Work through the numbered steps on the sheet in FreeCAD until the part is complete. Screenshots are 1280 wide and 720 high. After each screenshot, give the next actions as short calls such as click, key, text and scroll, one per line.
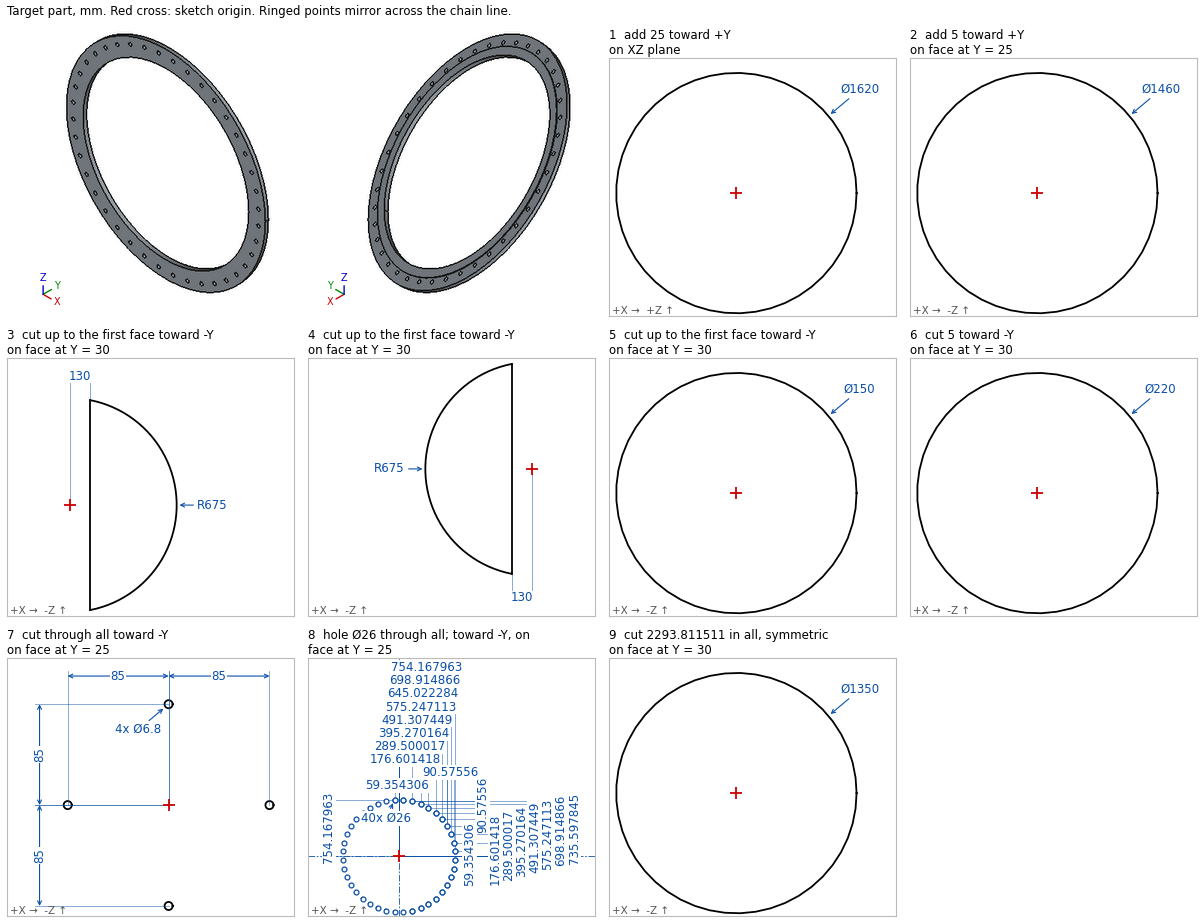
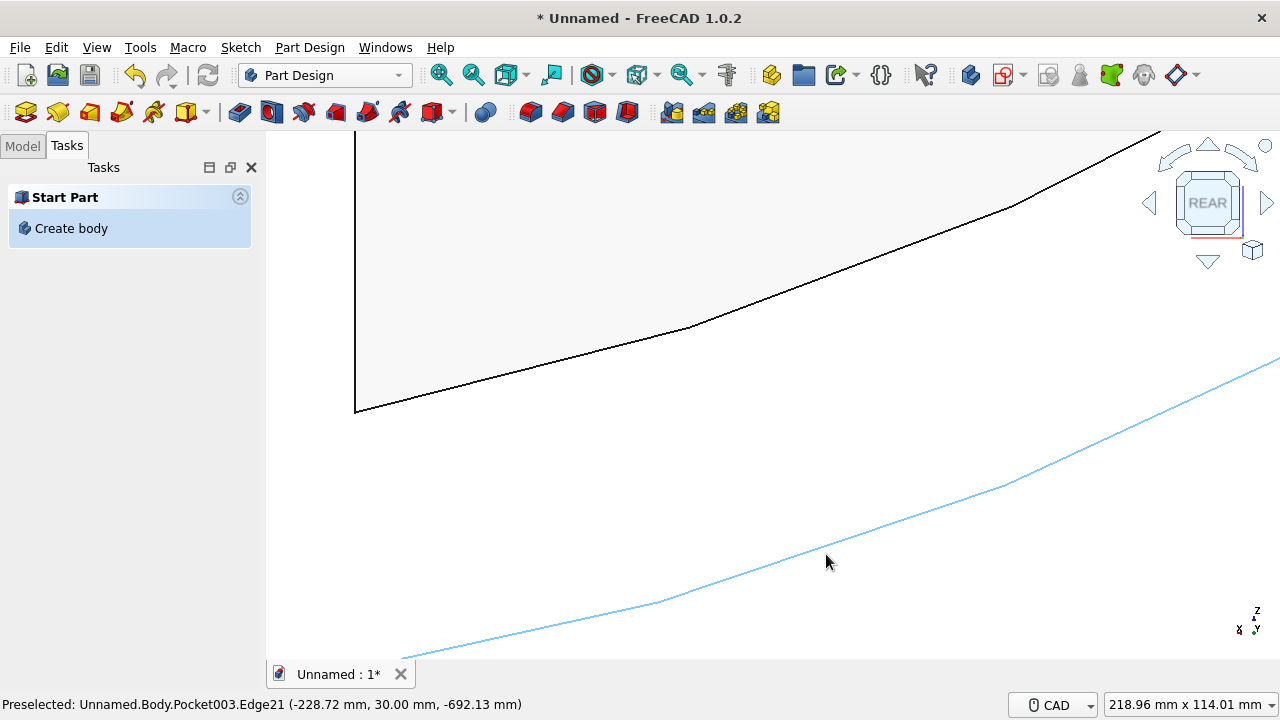
click(825, 559)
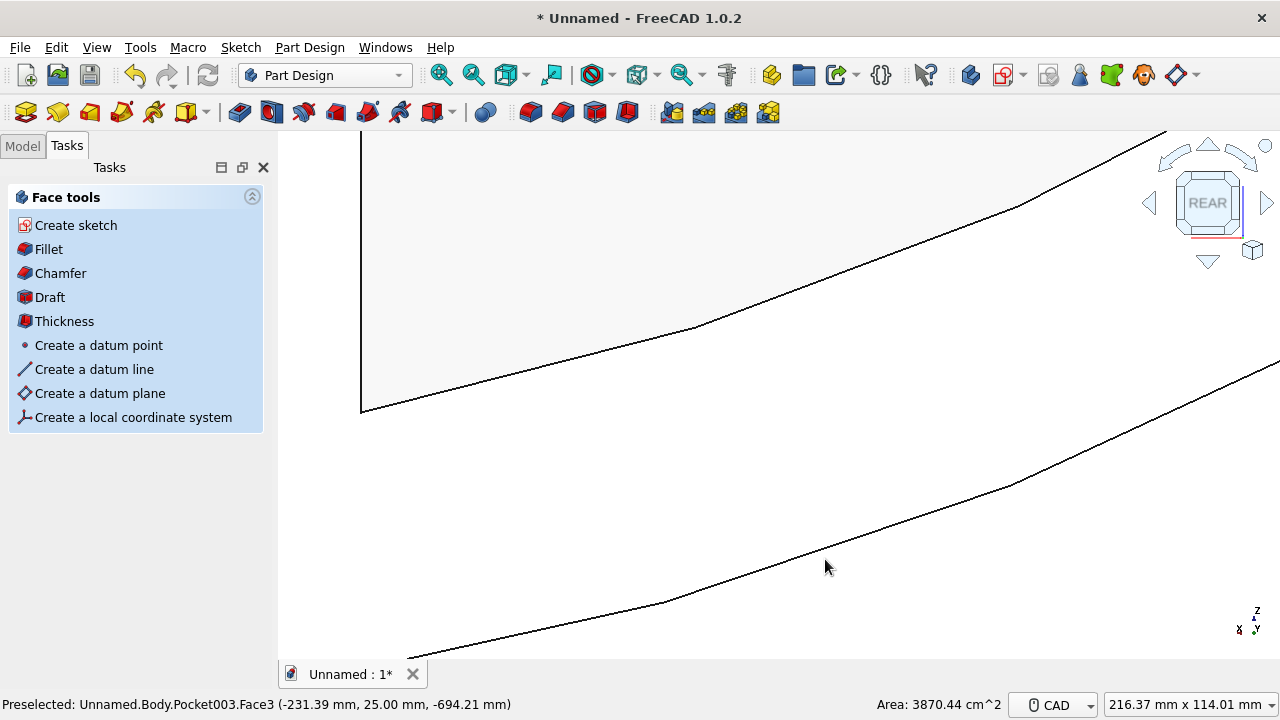
click(1004, 76)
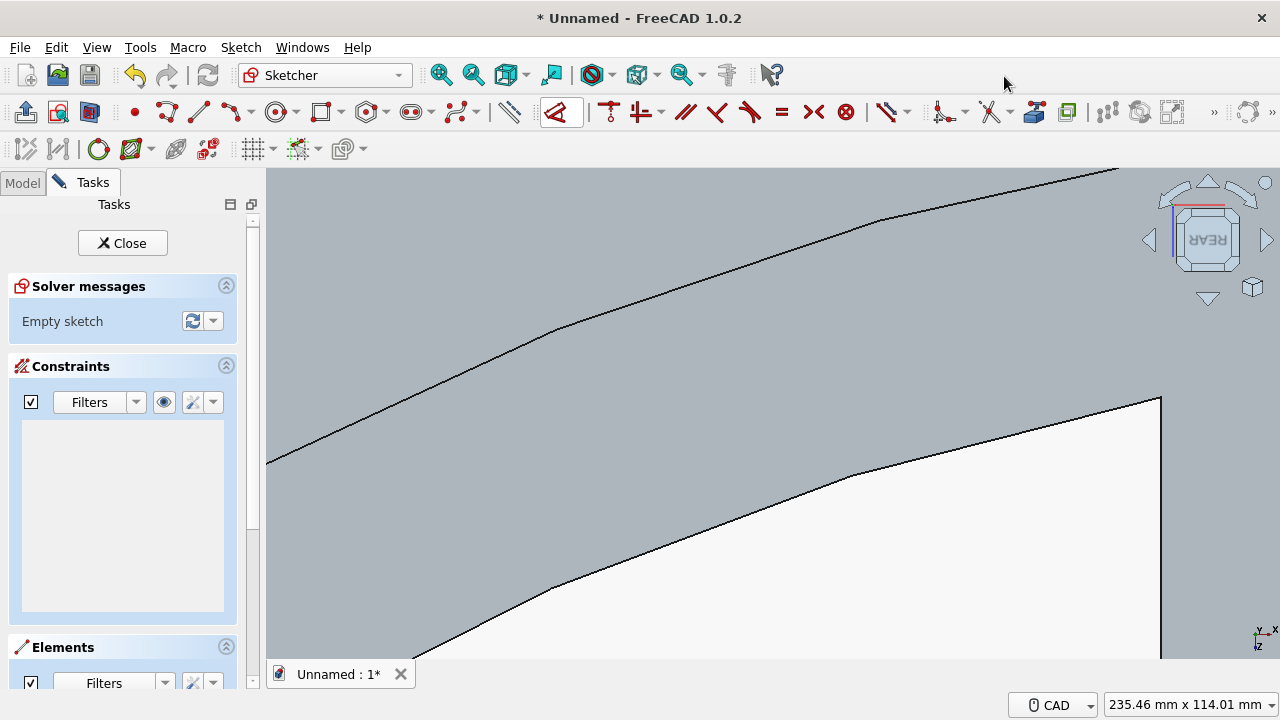
click(90, 112)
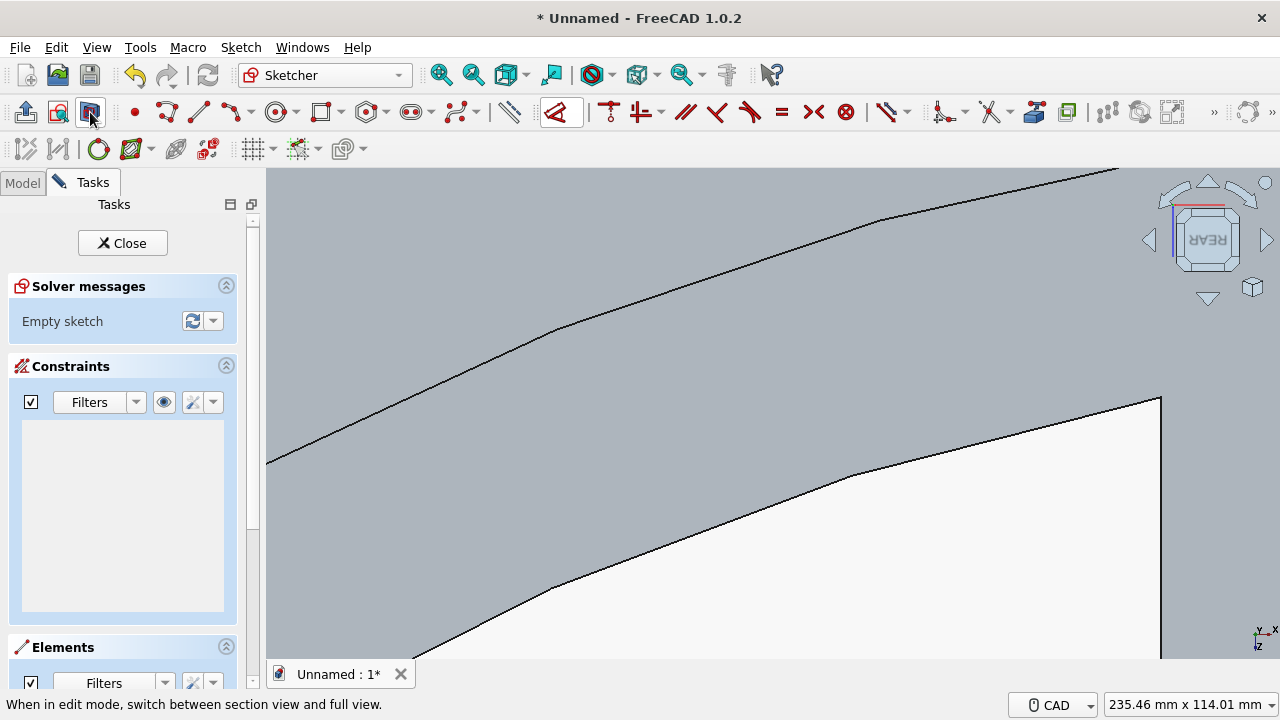
scroll(704, 414, down, 5)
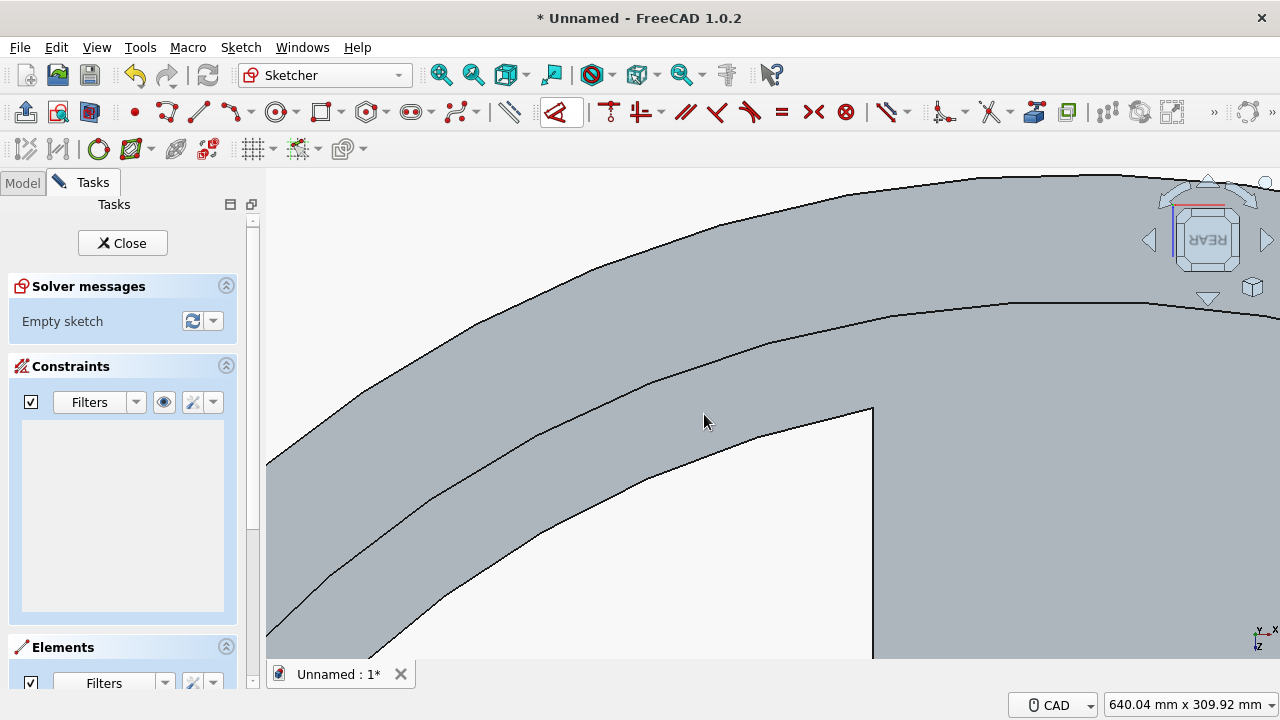
scroll(704, 414, down, 5)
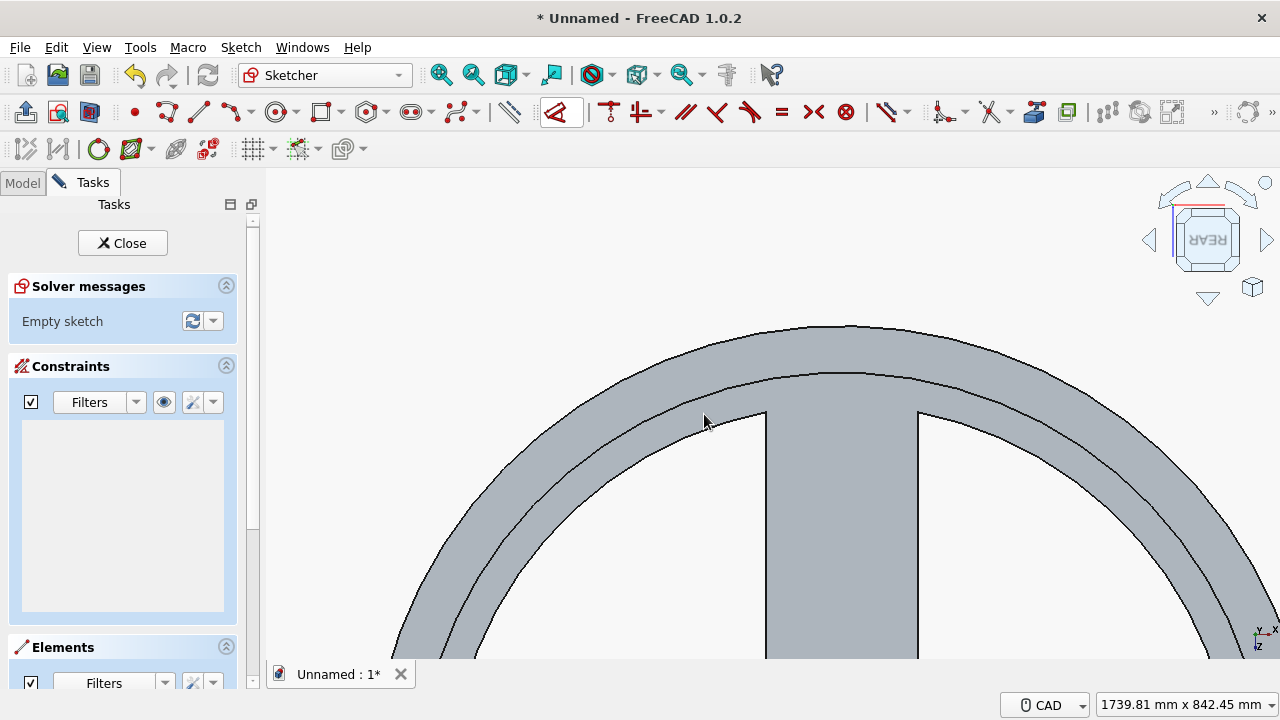
scroll(704, 414, down, 5)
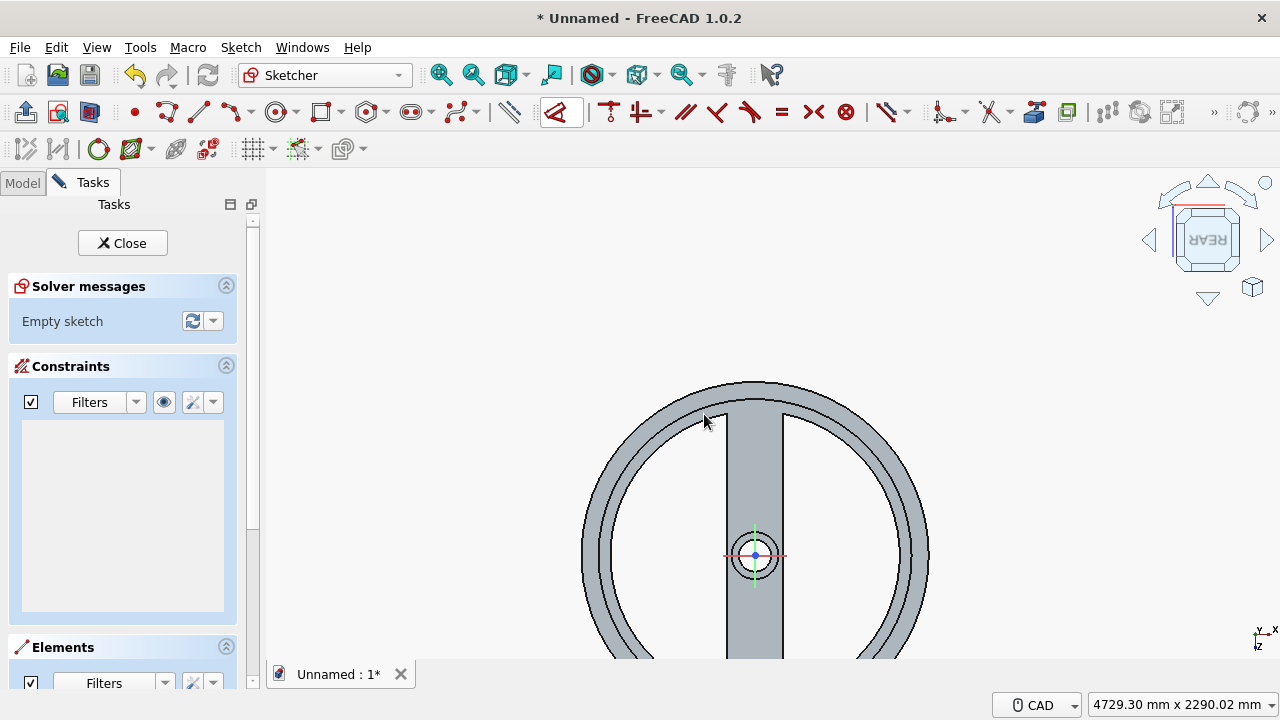
scroll(763, 578, up, 10)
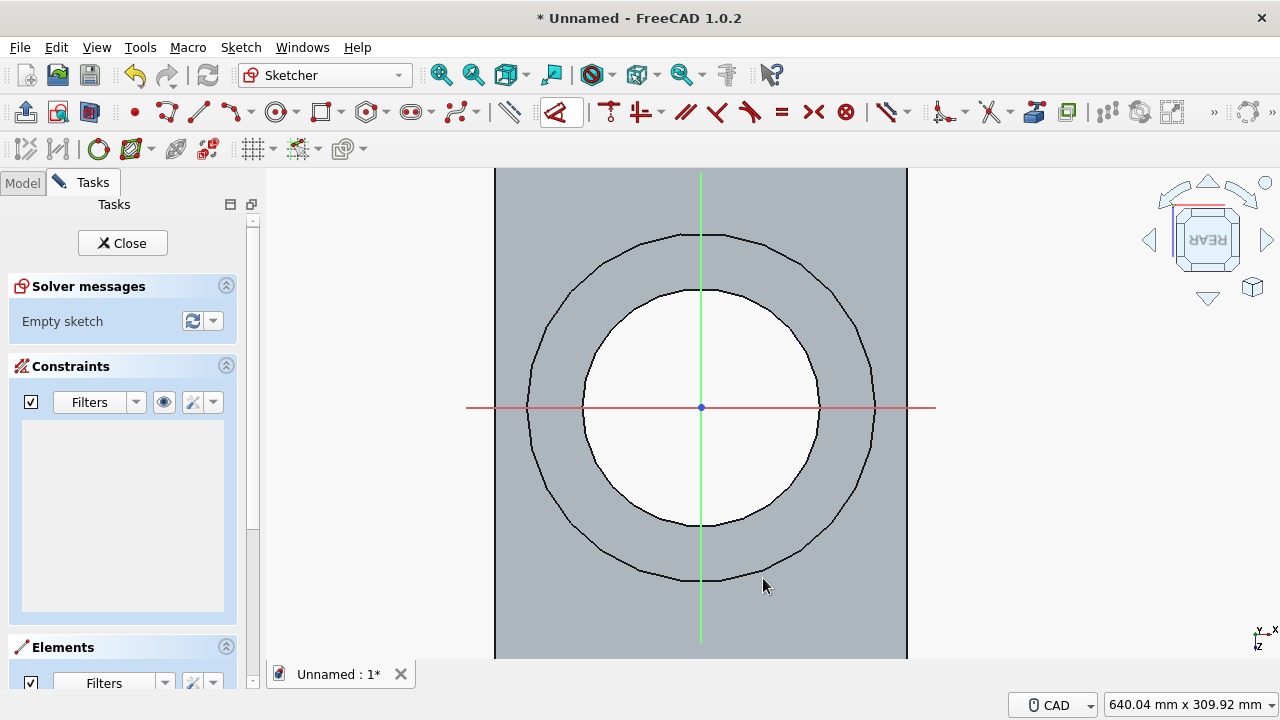
click(276, 112)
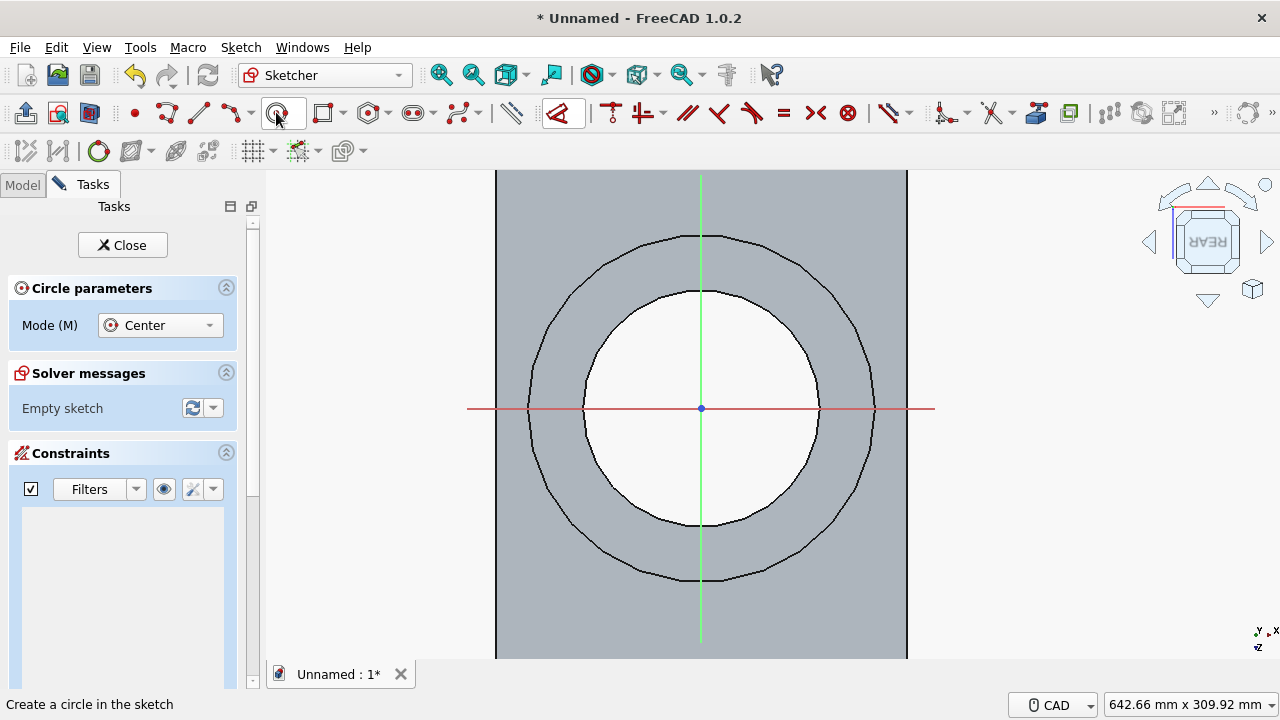
scroll(701, 274, up, 8)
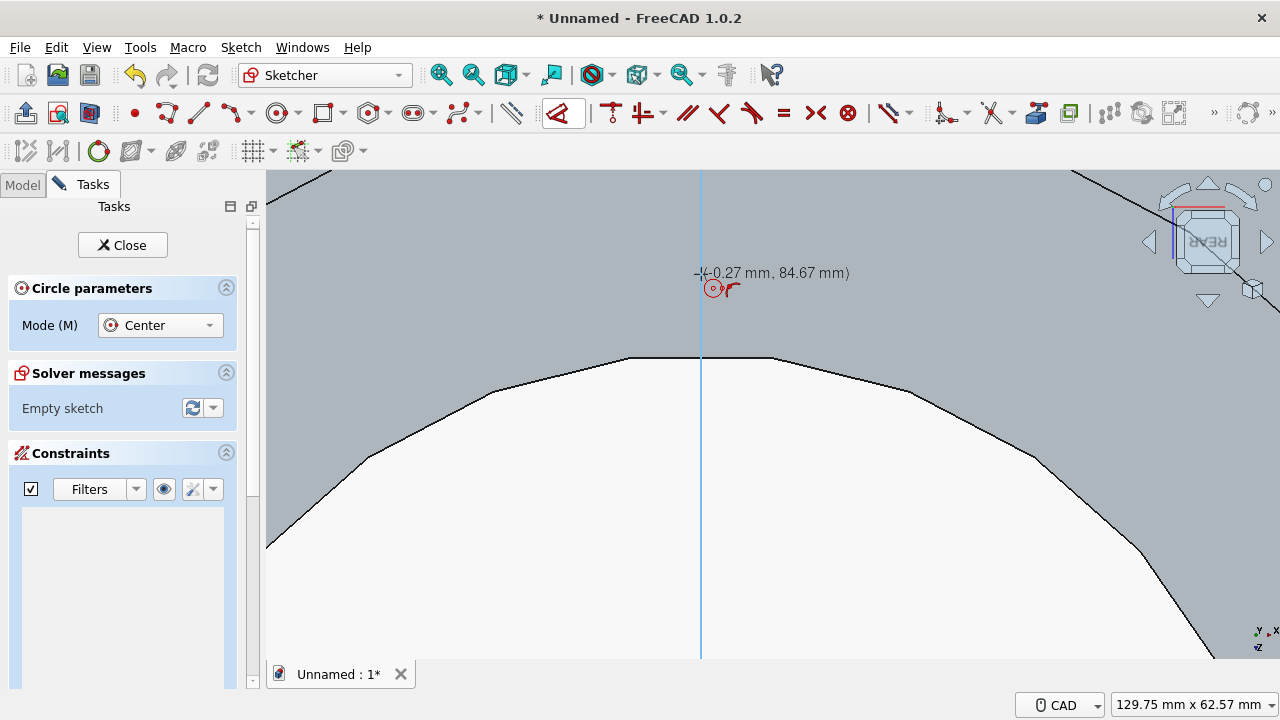
scroll(705, 282, down, 8)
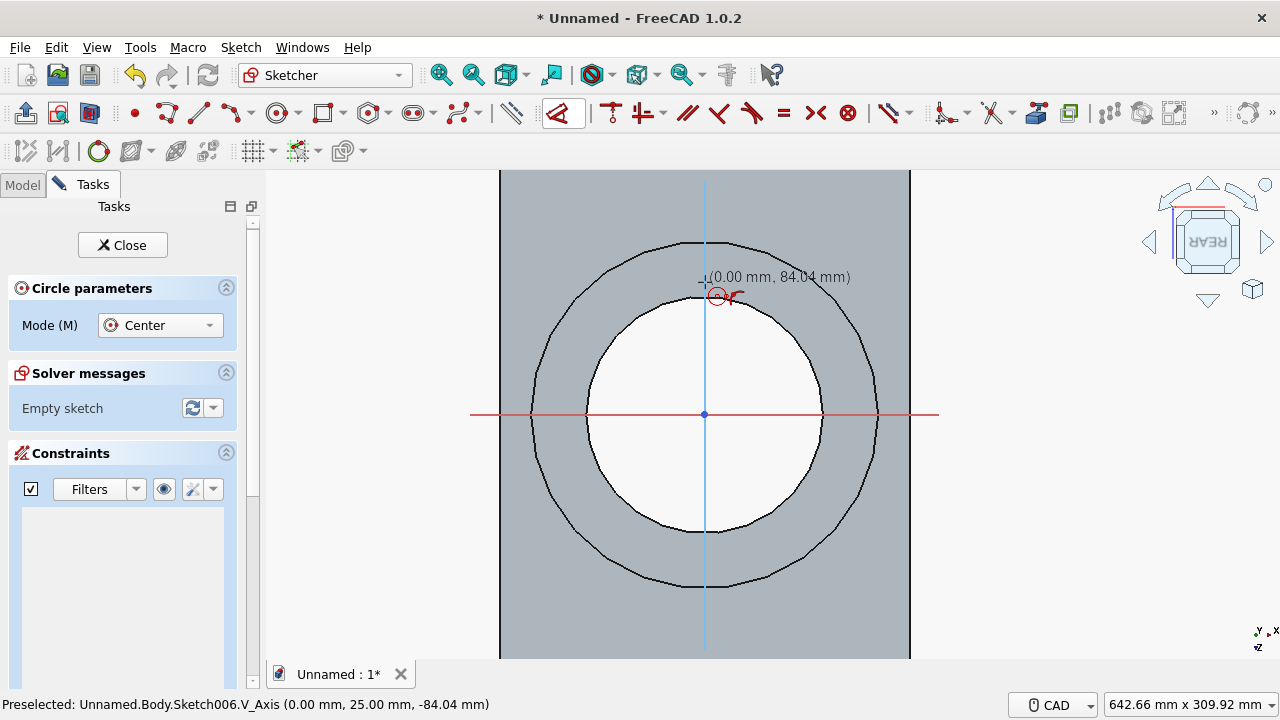
click(705, 281)